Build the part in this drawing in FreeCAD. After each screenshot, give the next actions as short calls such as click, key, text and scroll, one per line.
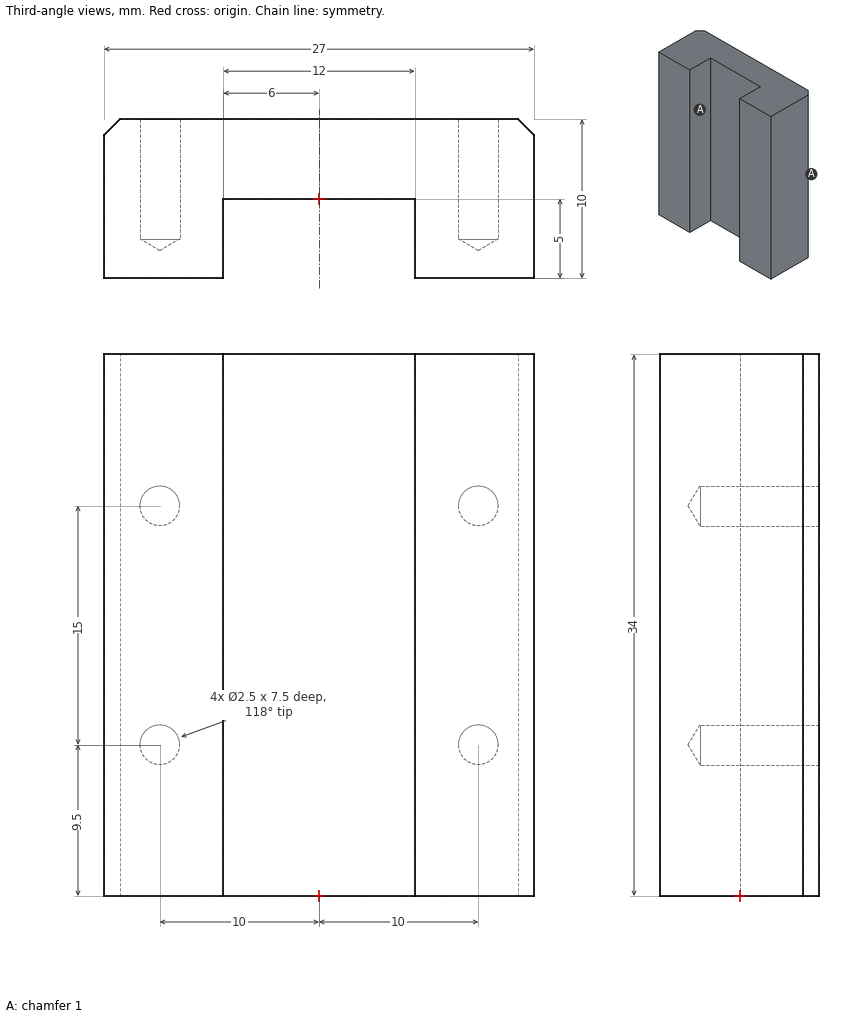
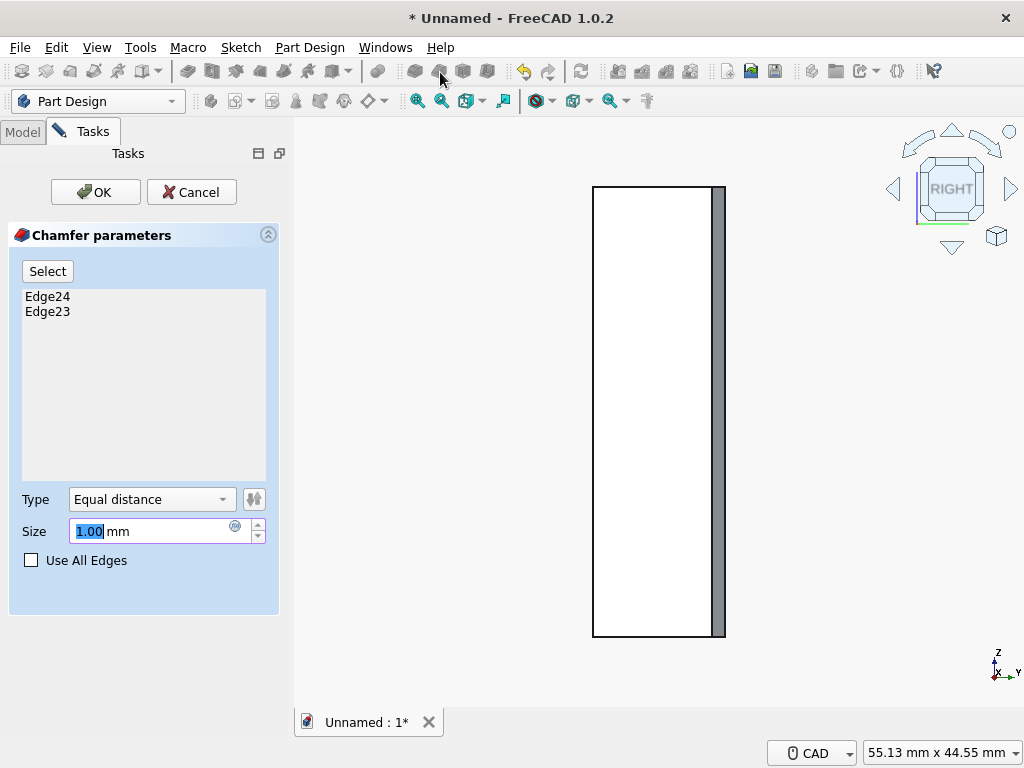
text(1)
key(Tab)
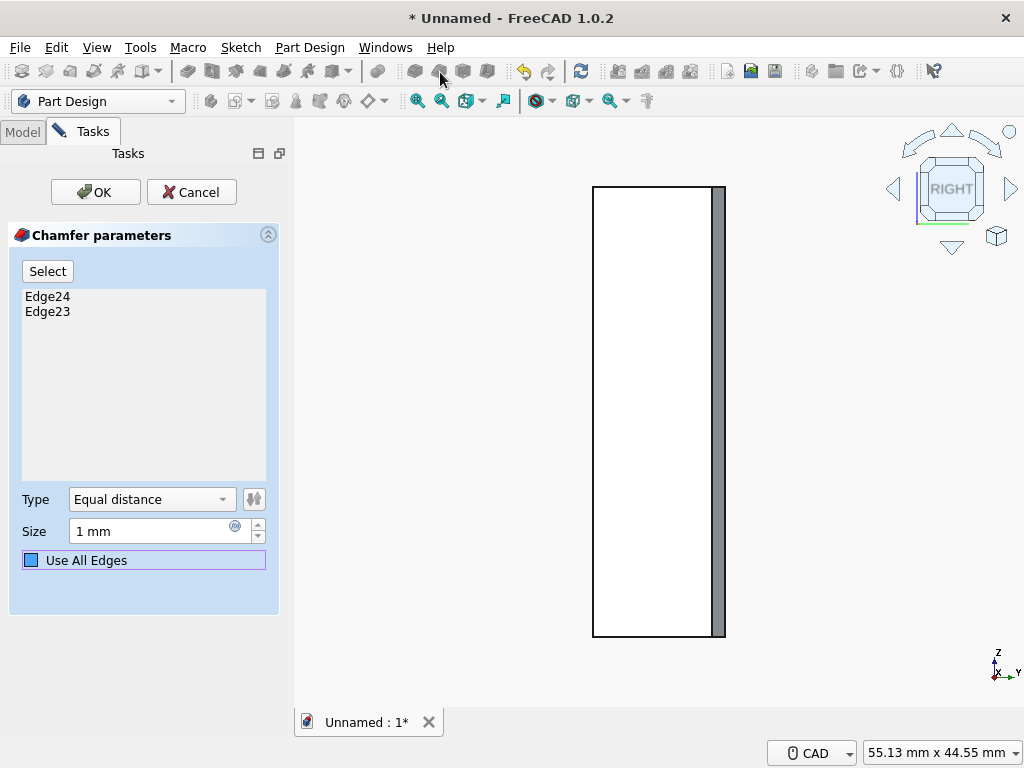
click(96, 192)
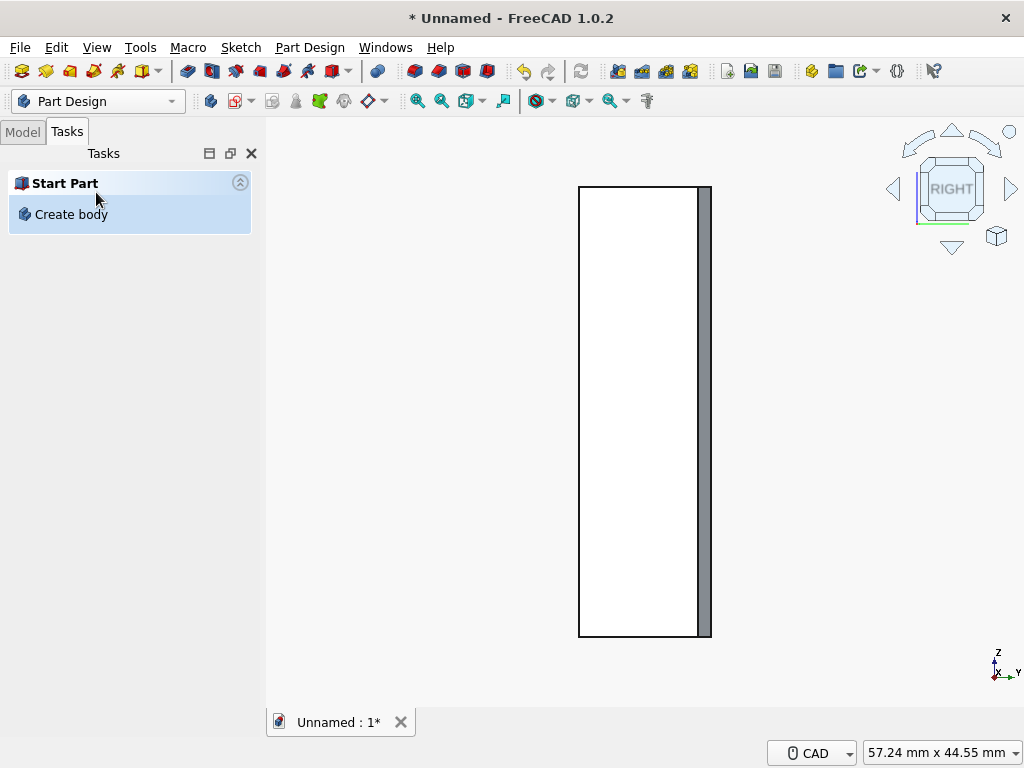
key(0)